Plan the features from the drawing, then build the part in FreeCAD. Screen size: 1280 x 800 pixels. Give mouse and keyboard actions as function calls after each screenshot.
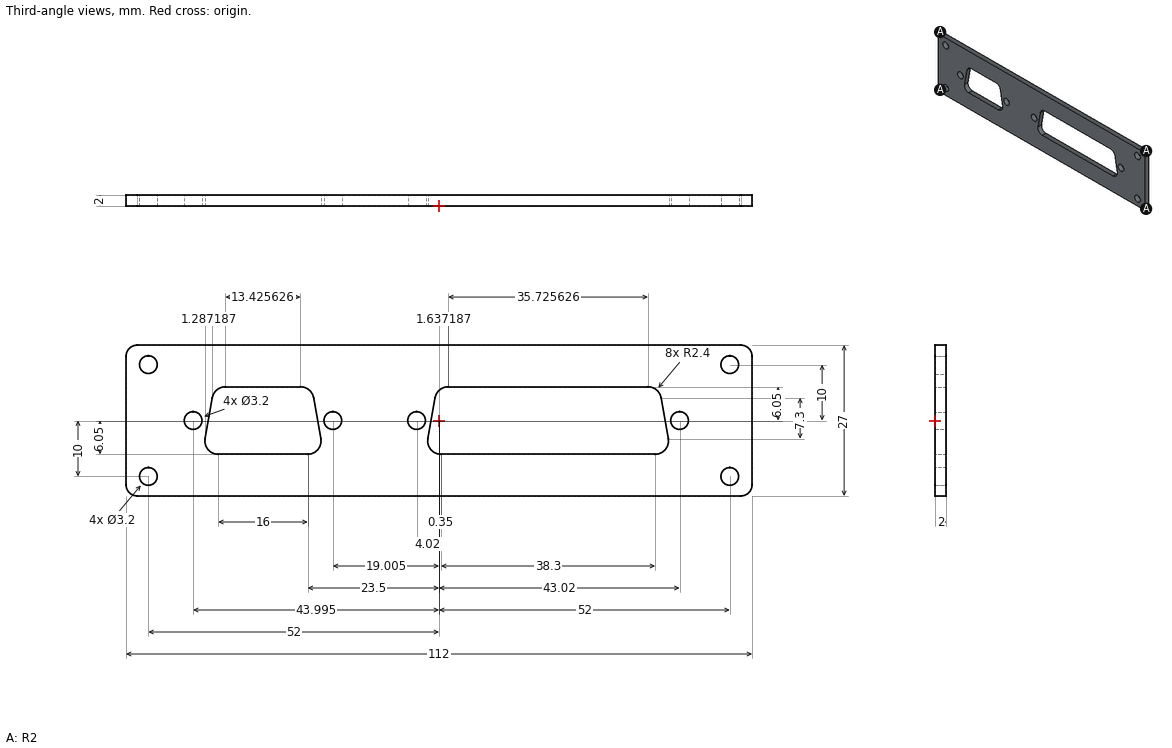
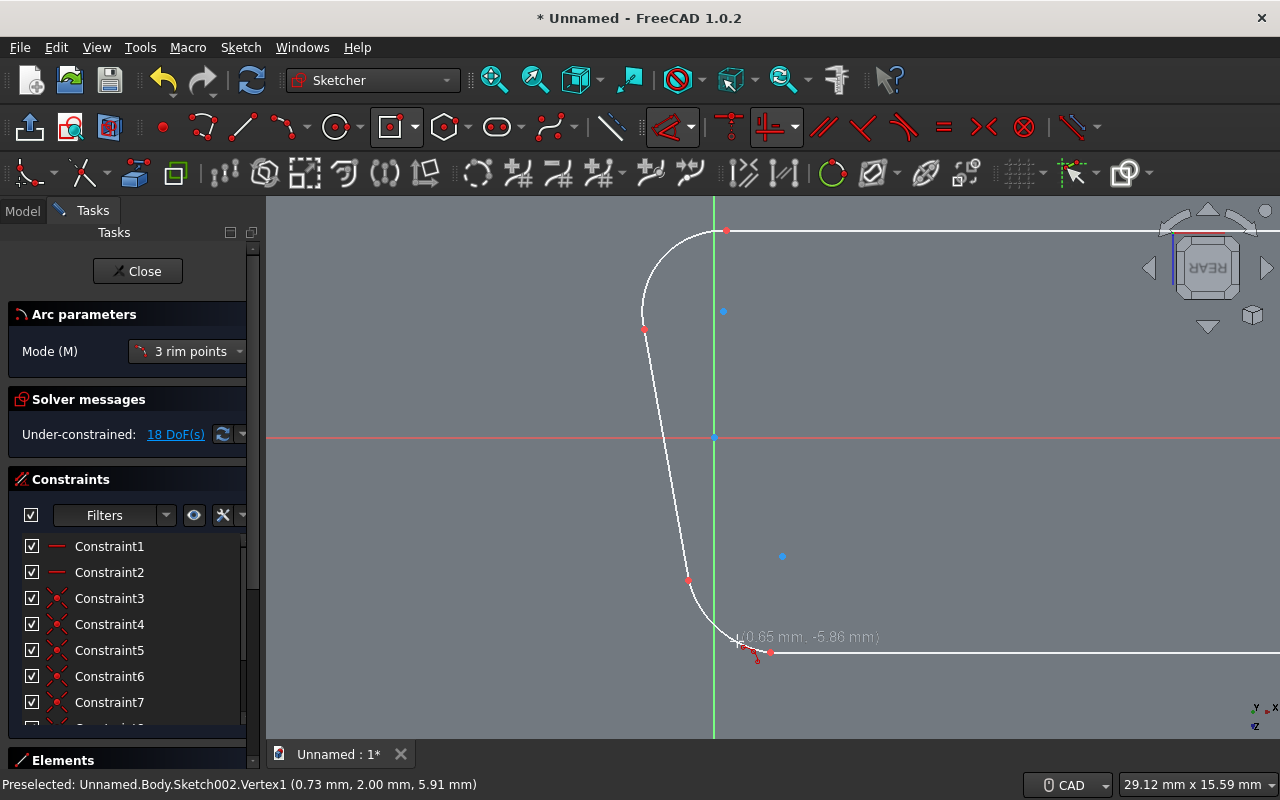
key(g)
key(l)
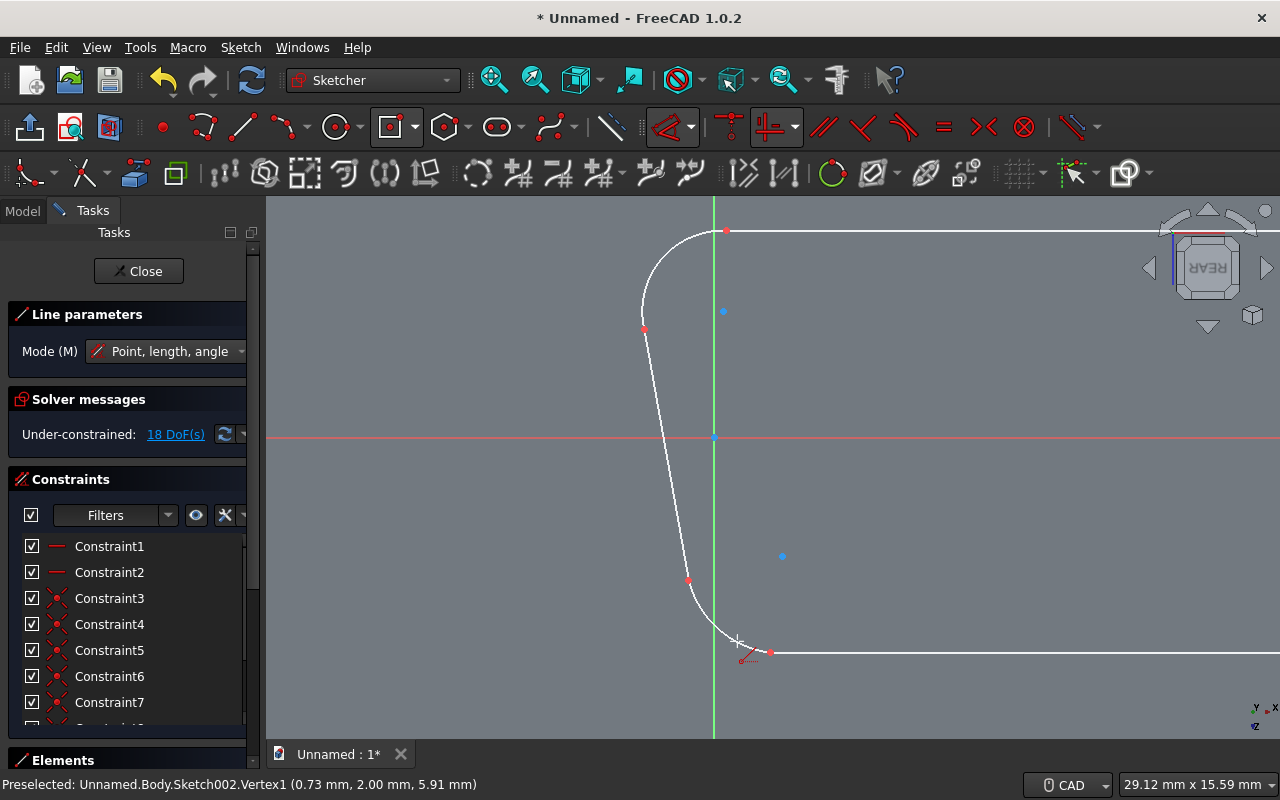
scroll(706, 475, down, 8)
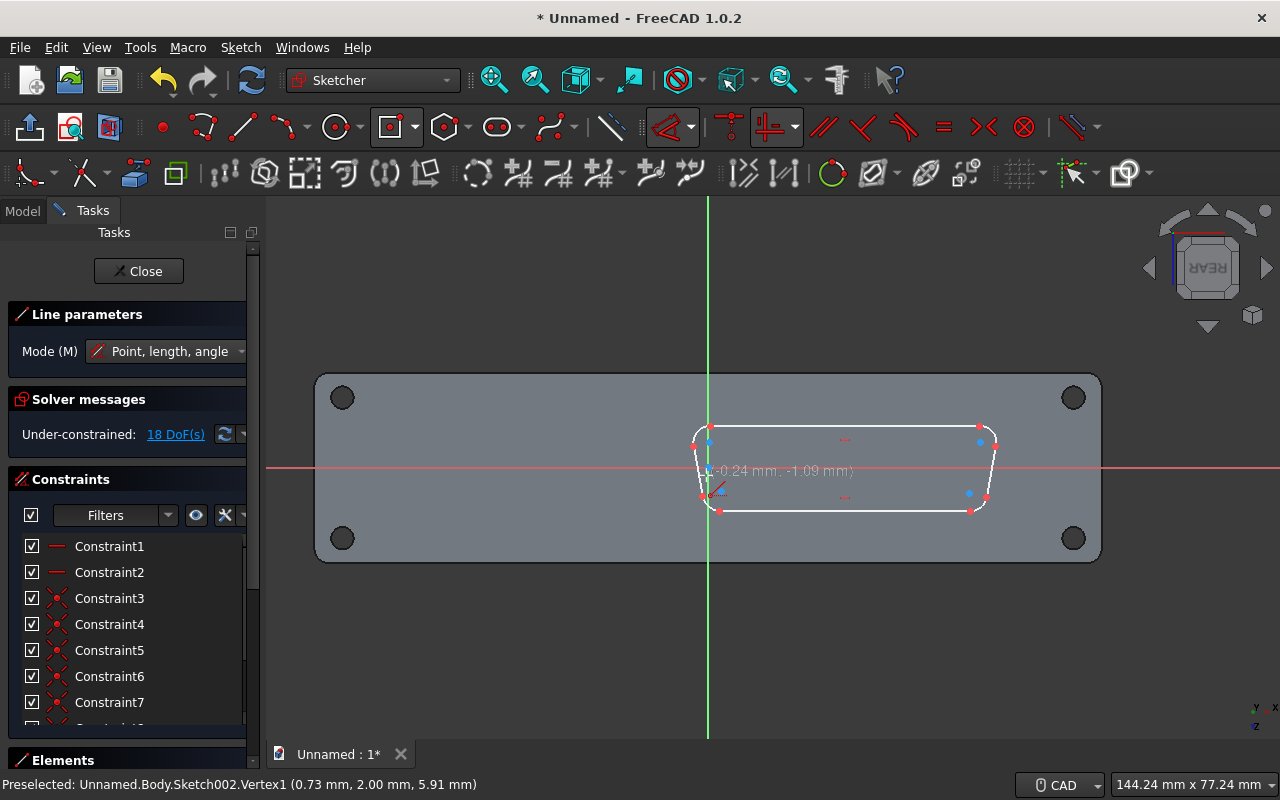
click(543, 425)
click(430, 425)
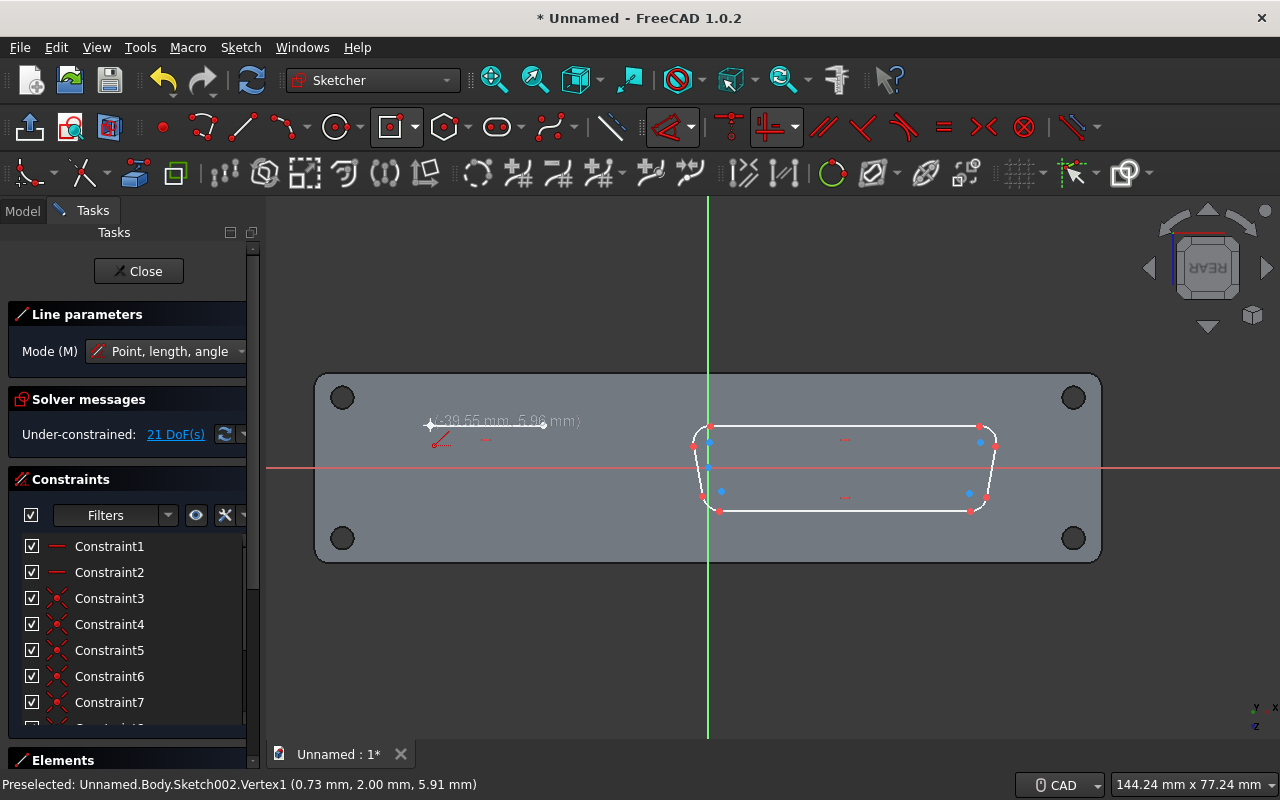
click(414, 445)
click(423, 497)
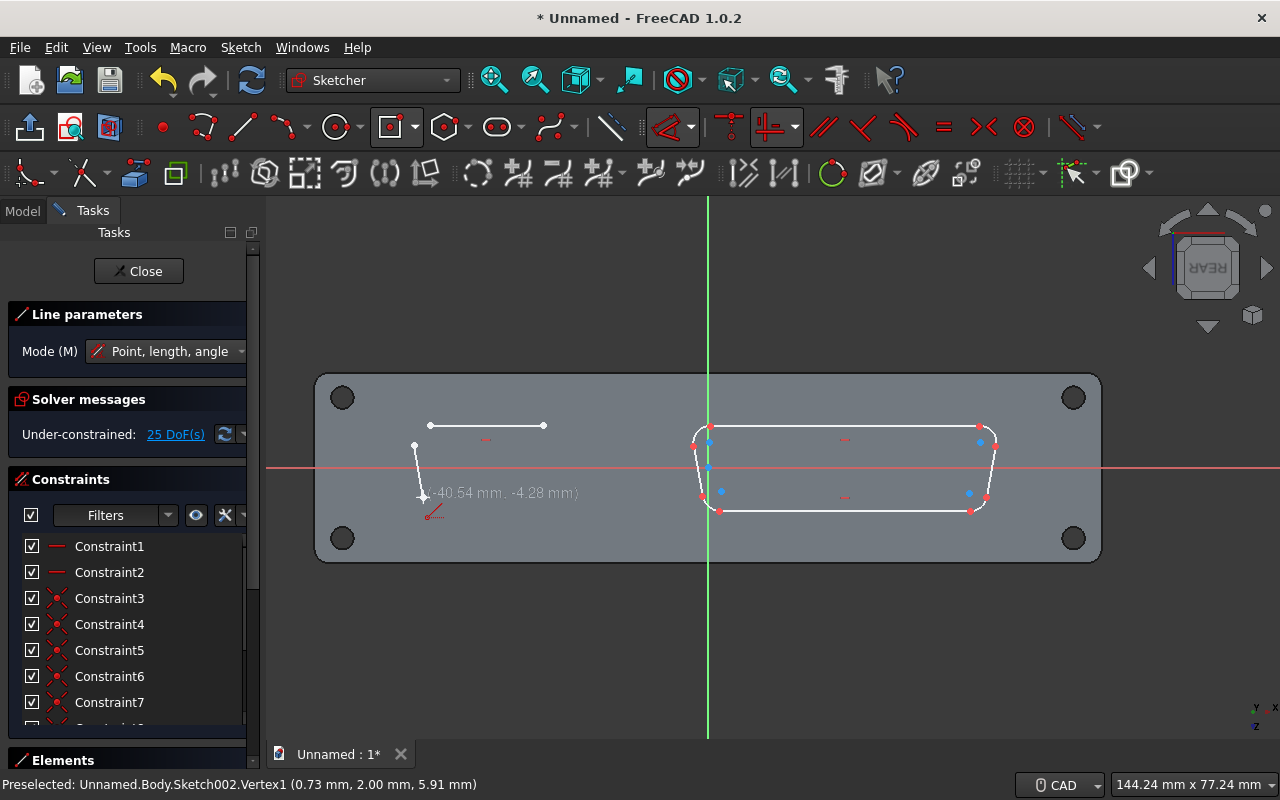
click(439, 510)
click(534, 510)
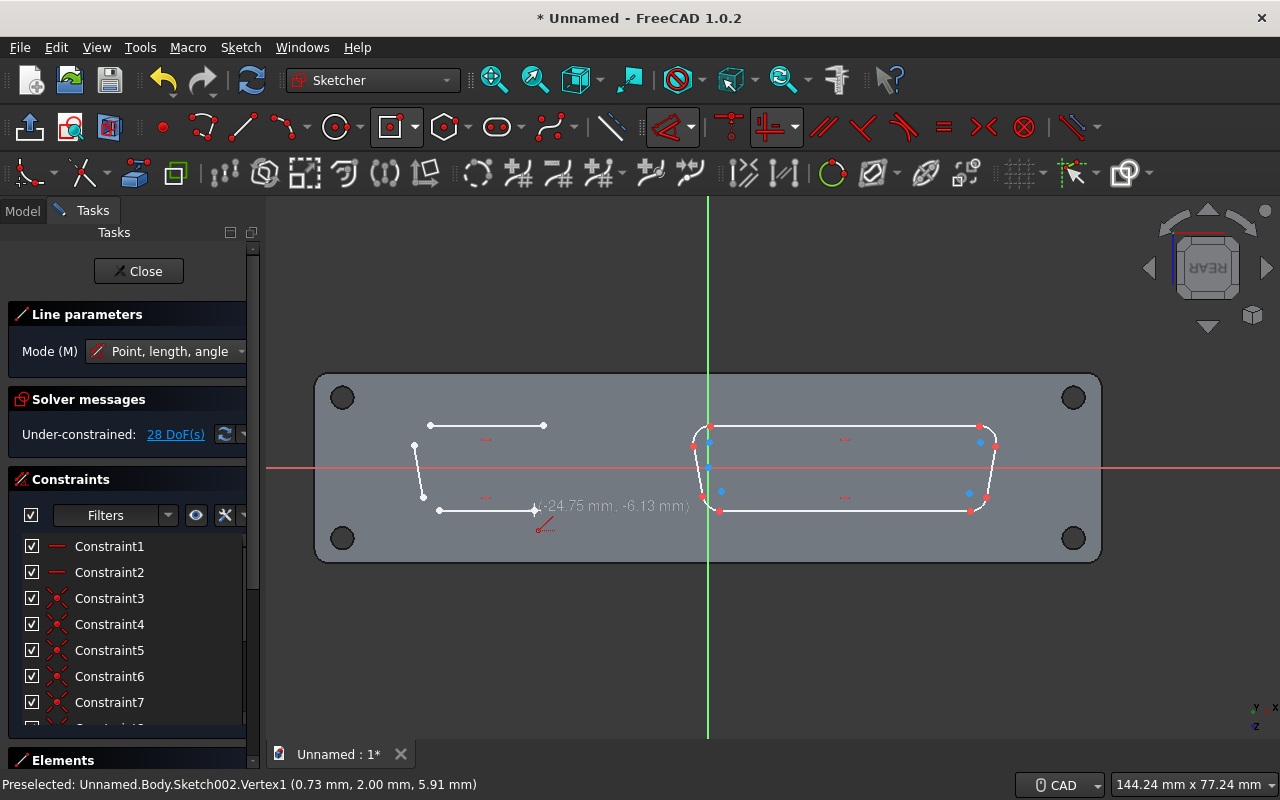
click(550, 497)
click(559, 445)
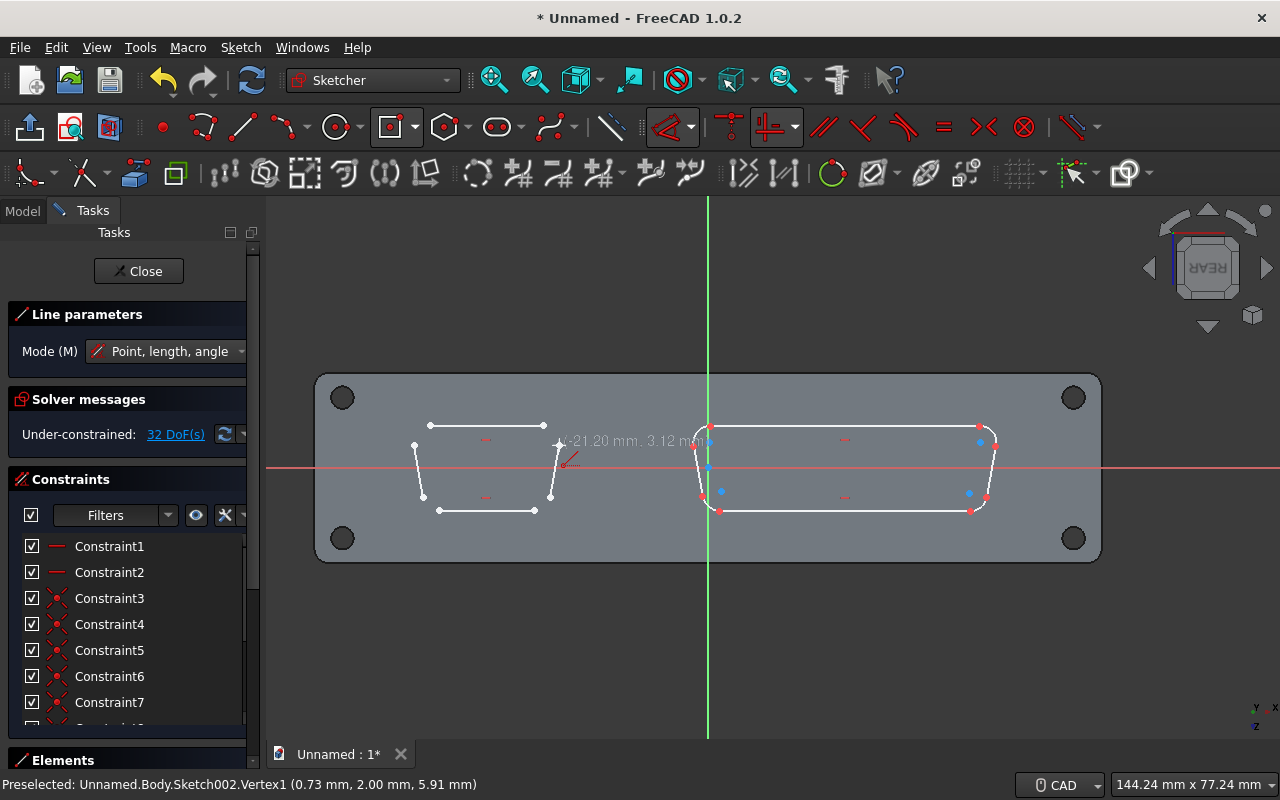
click(284, 128)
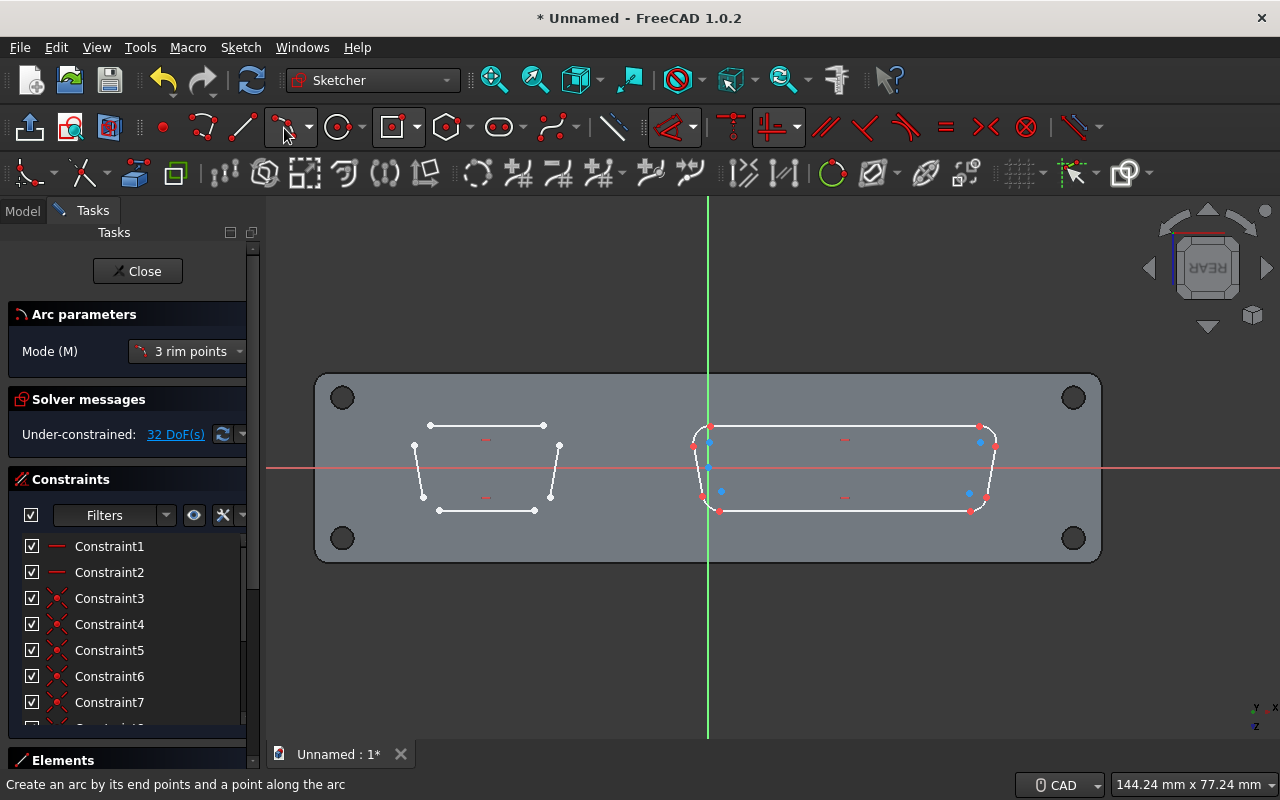
click(430, 426)
click(414, 446)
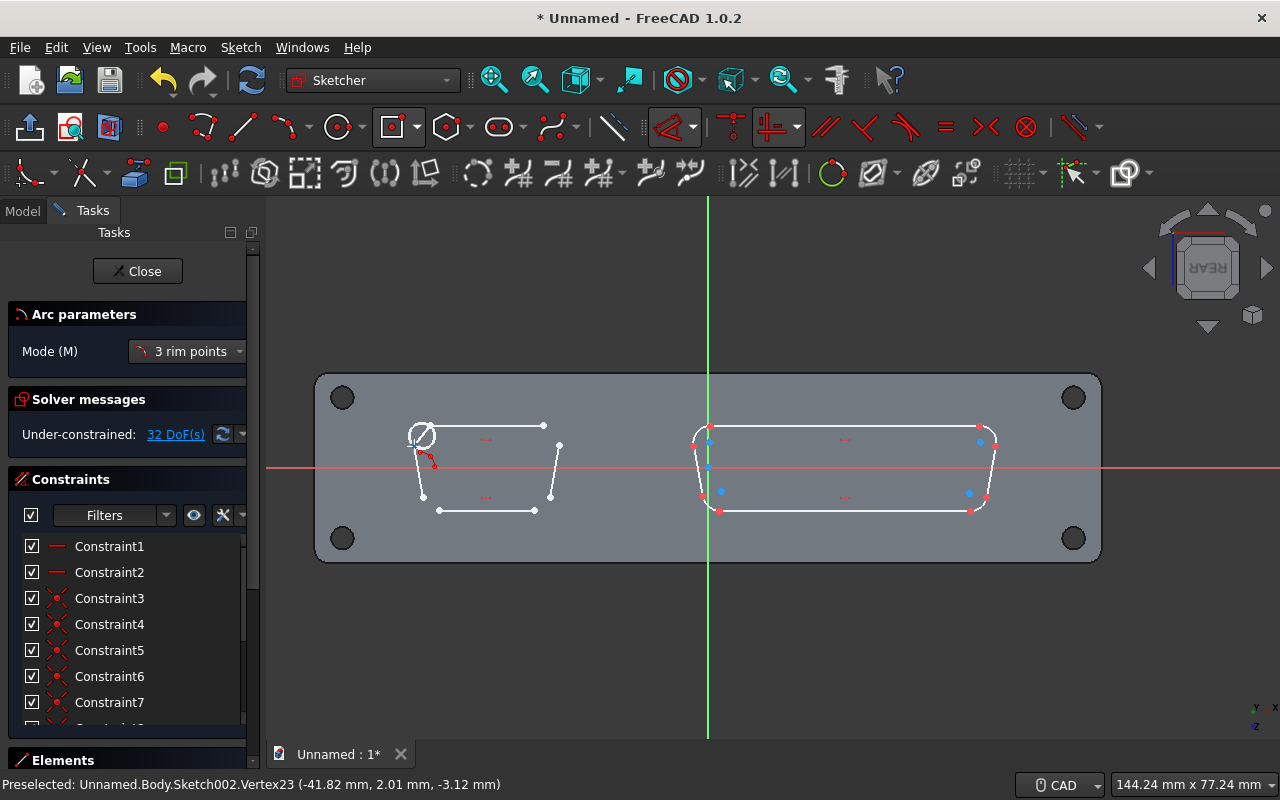
scroll(417, 431, up, 5)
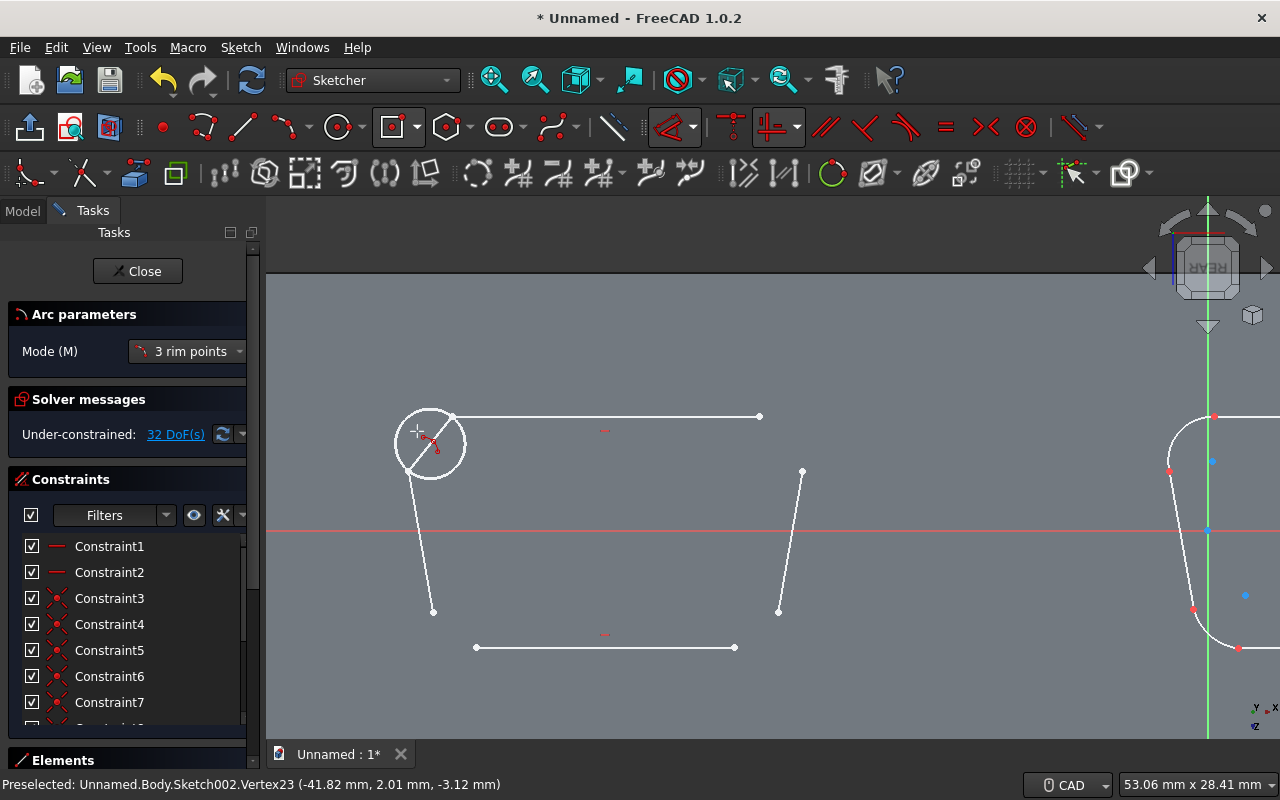
click(418, 431)